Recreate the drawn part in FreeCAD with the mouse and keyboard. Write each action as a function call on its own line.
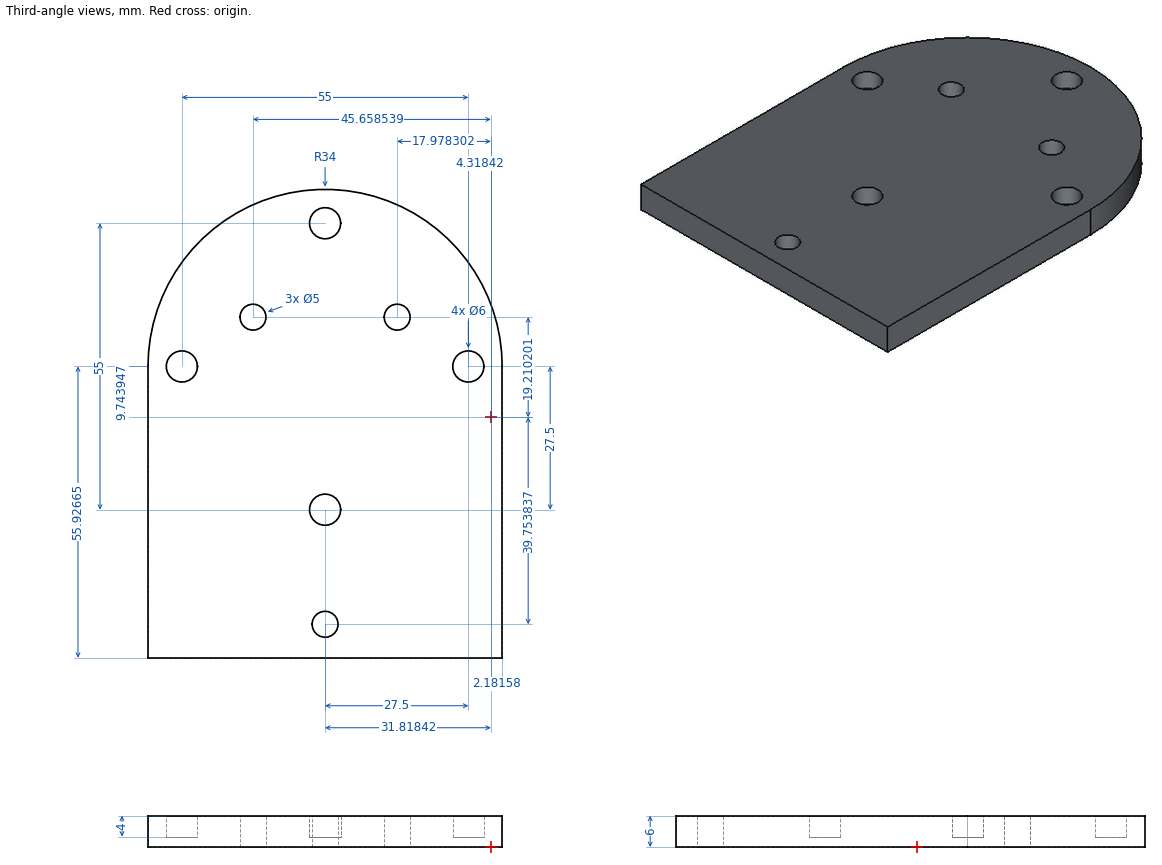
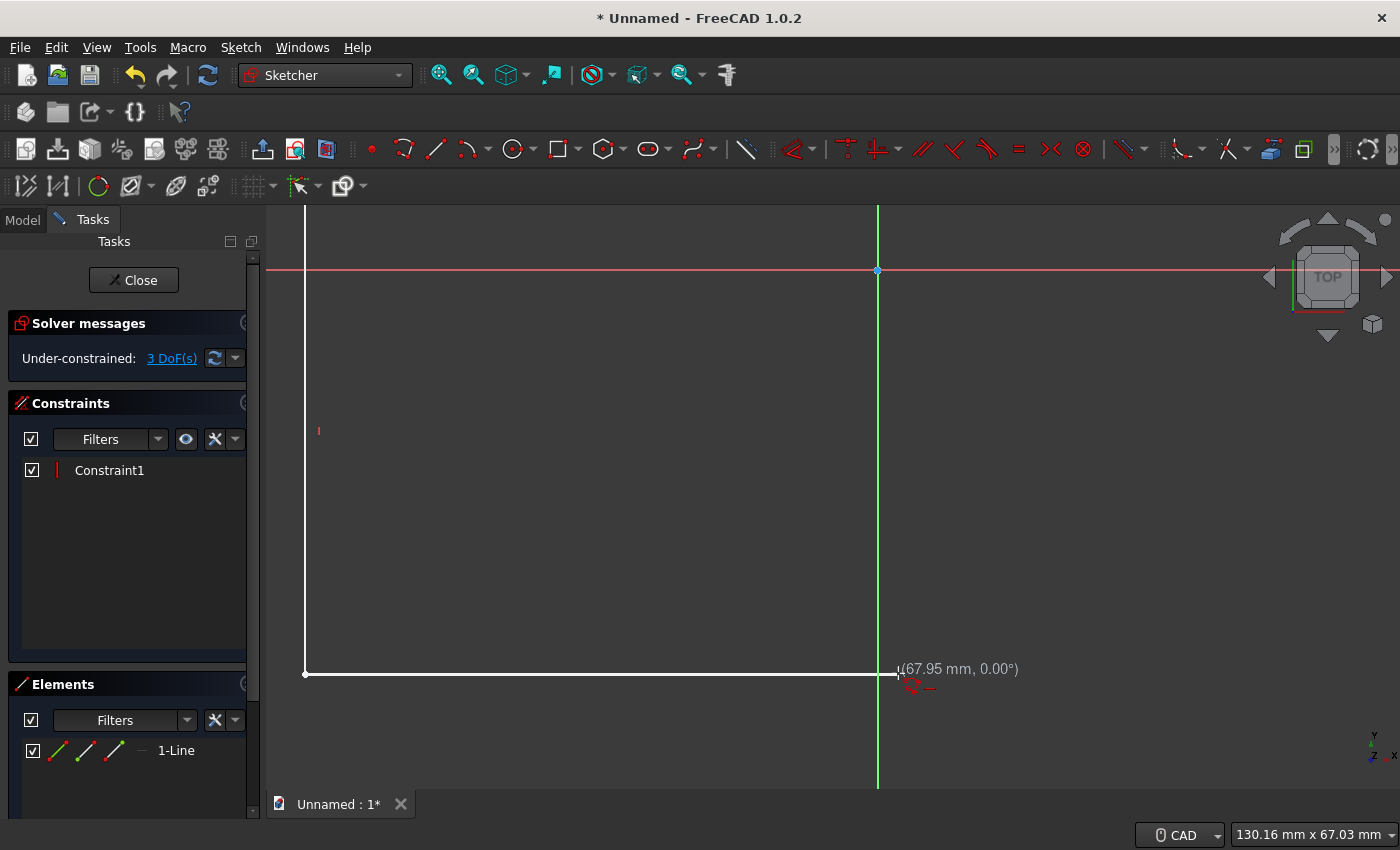
click(897, 672)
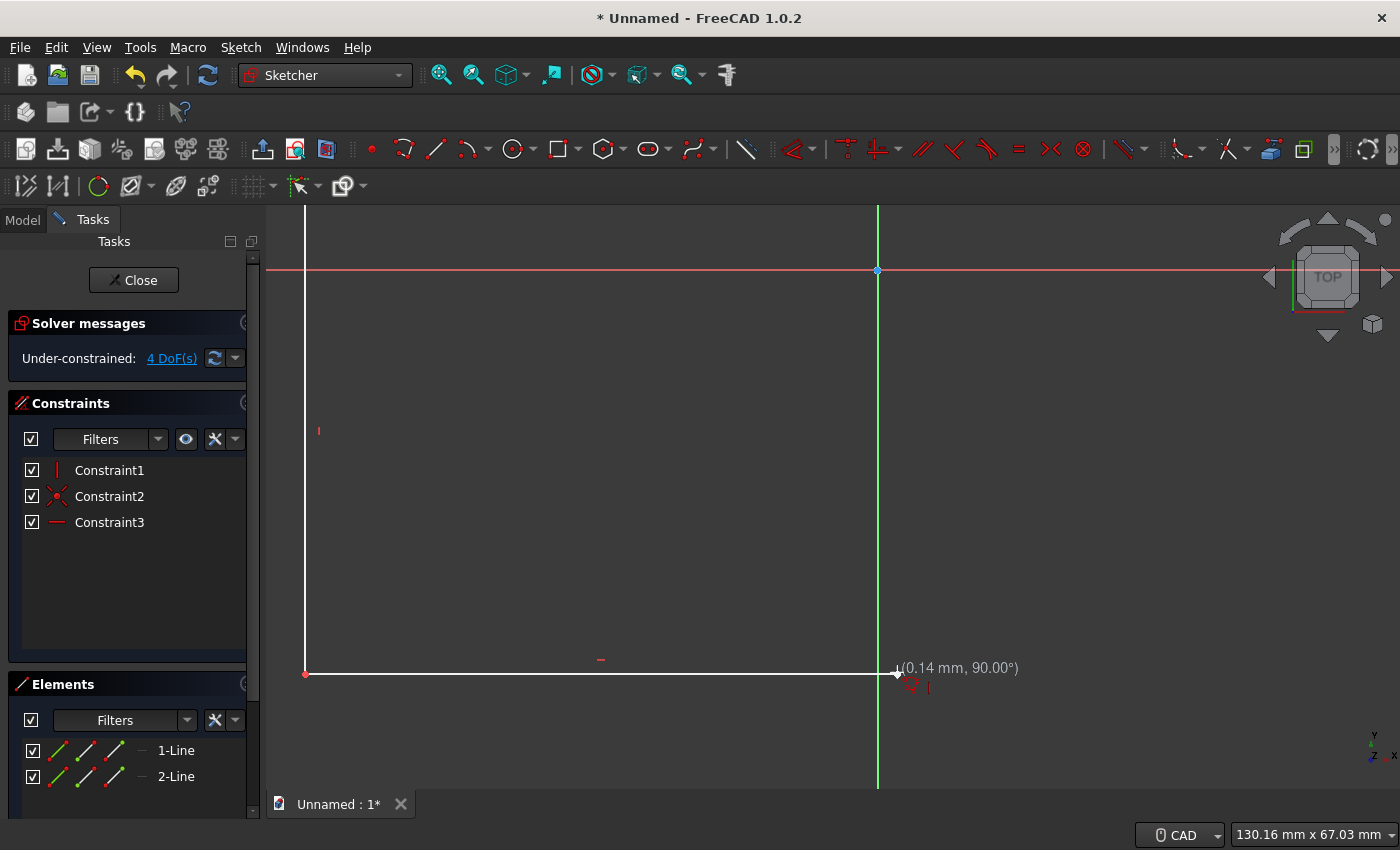
scroll(898, 673, down, 4)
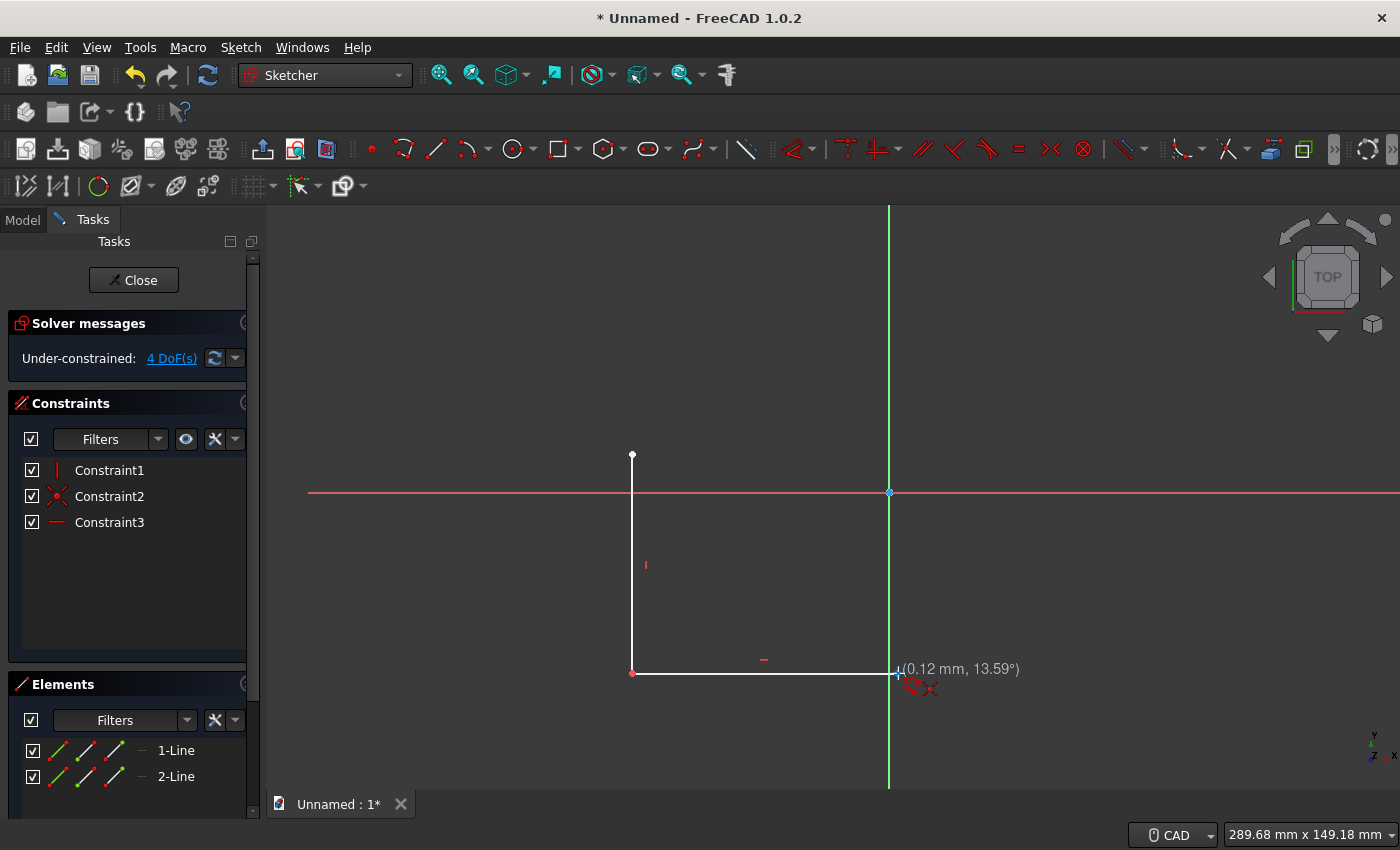
scroll(898, 454, up, 4)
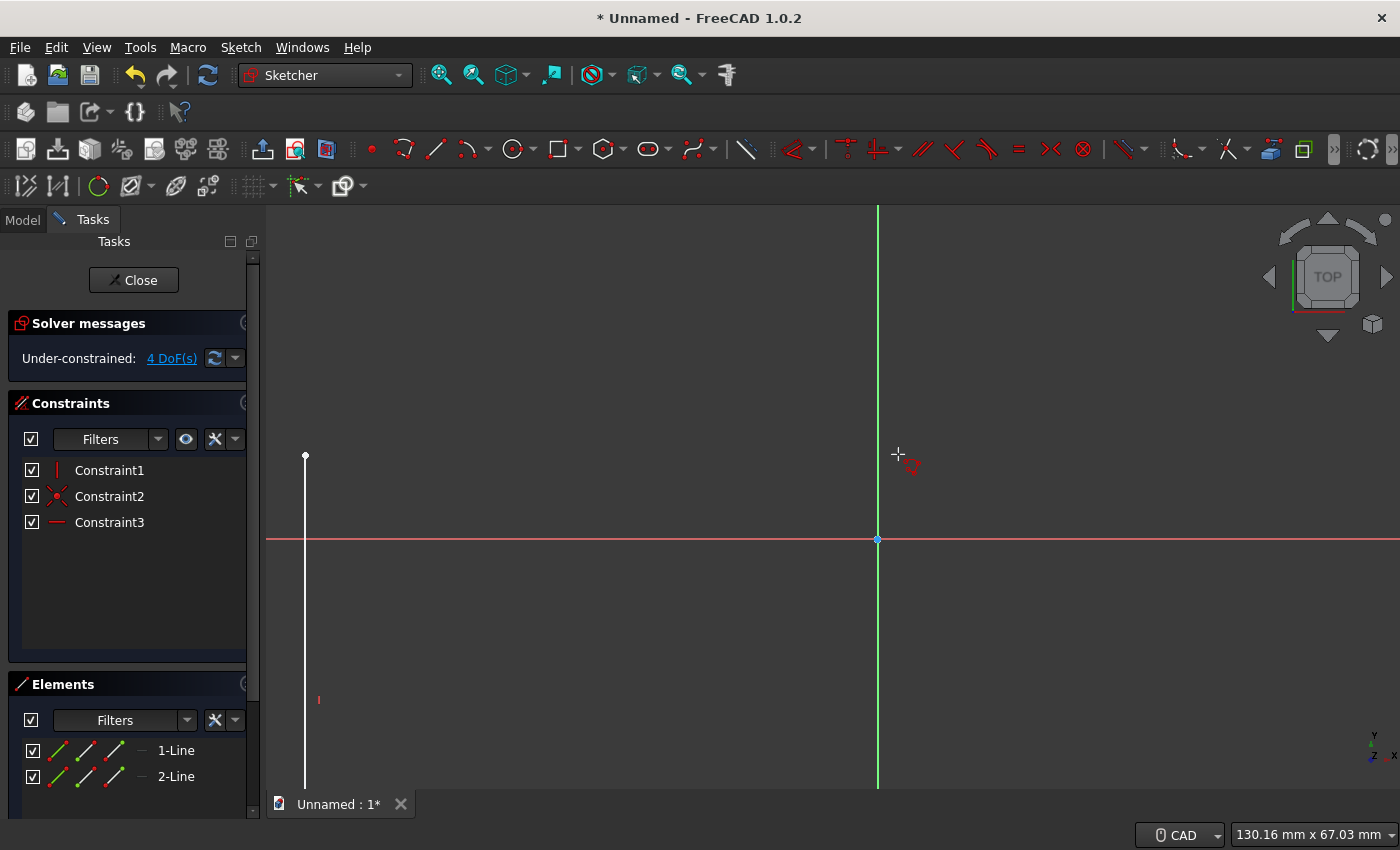
click(897, 454)
right_click(897, 454)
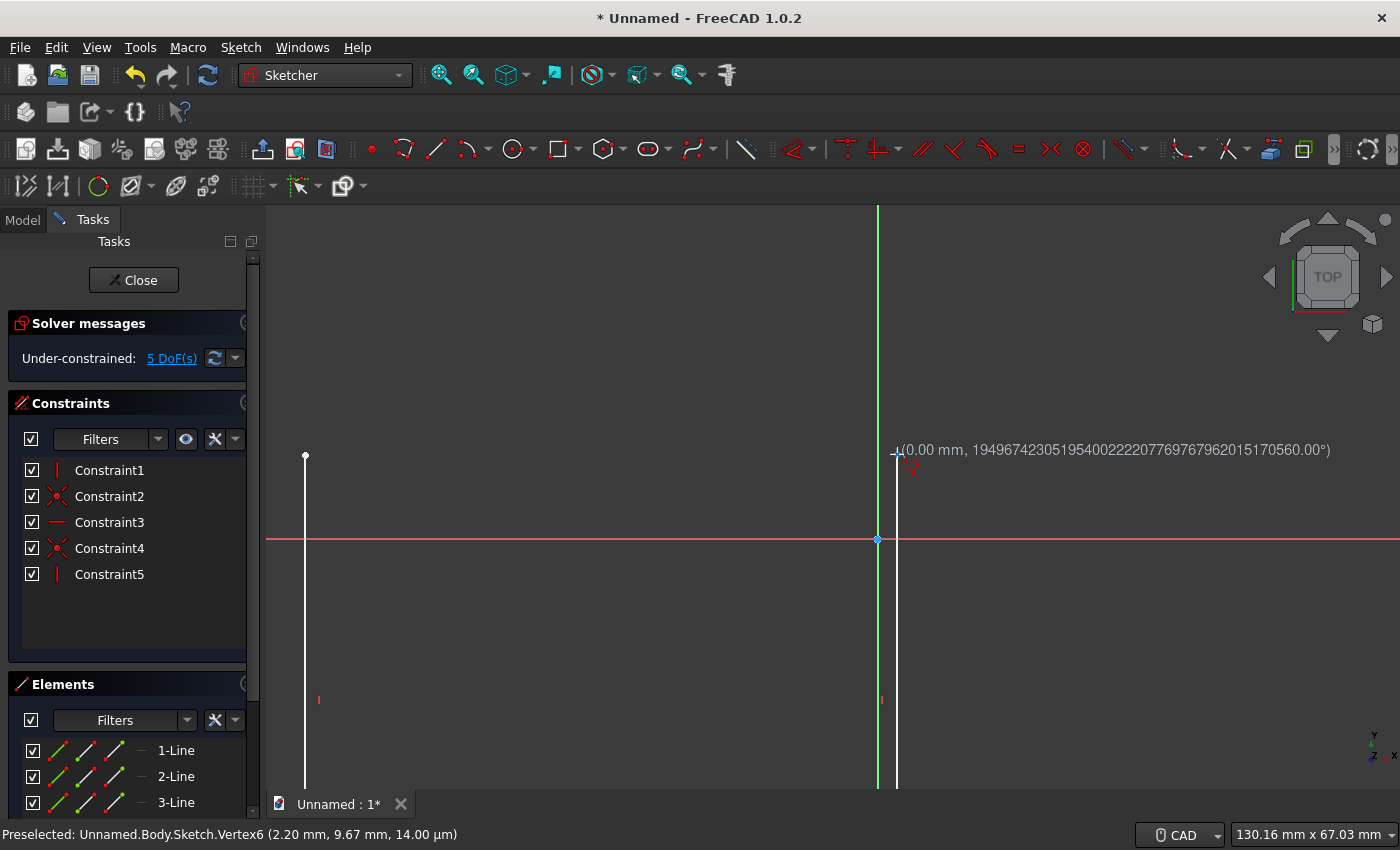
key(g)
key(3)
key(a)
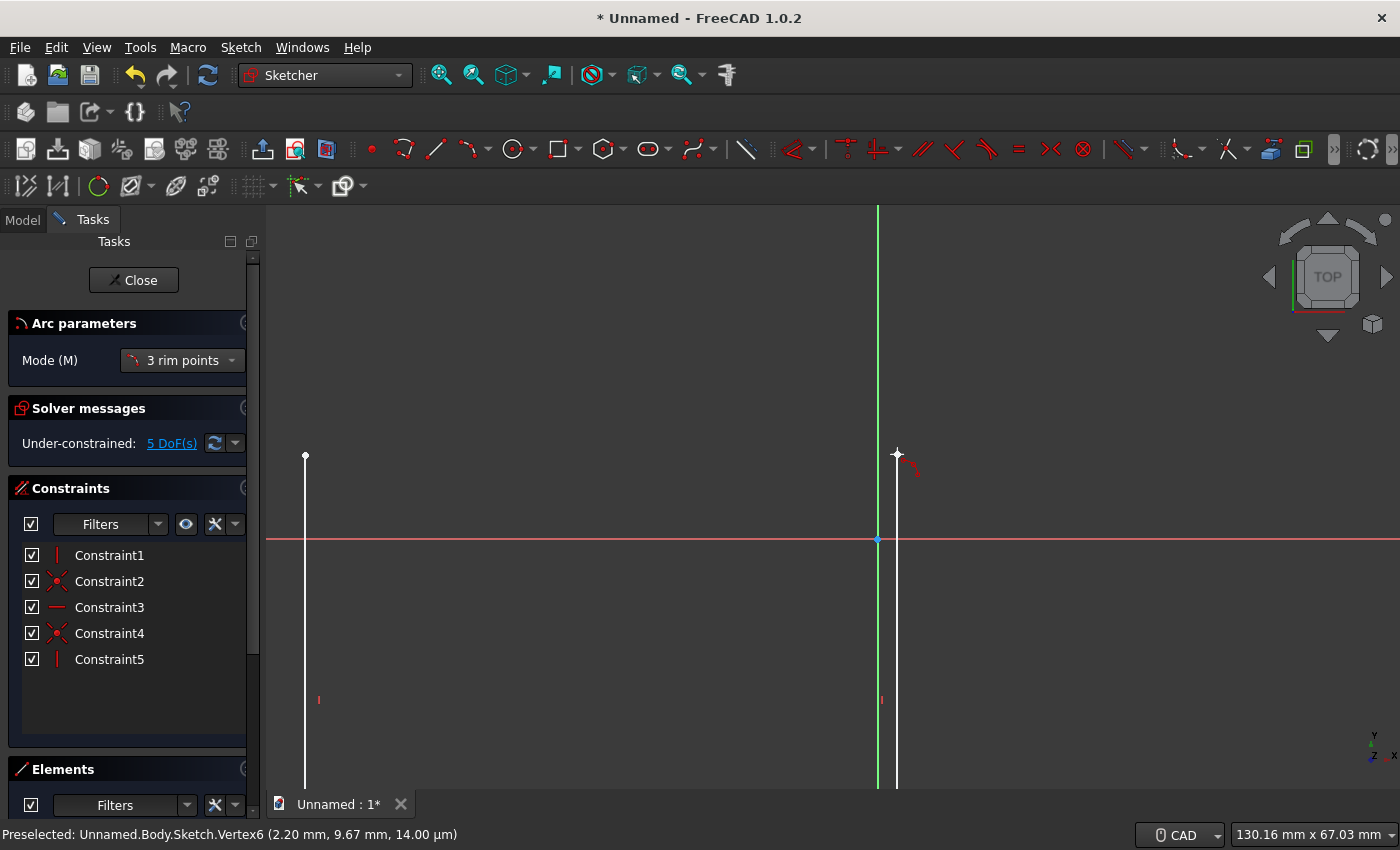
click(897, 455)
click(305, 456)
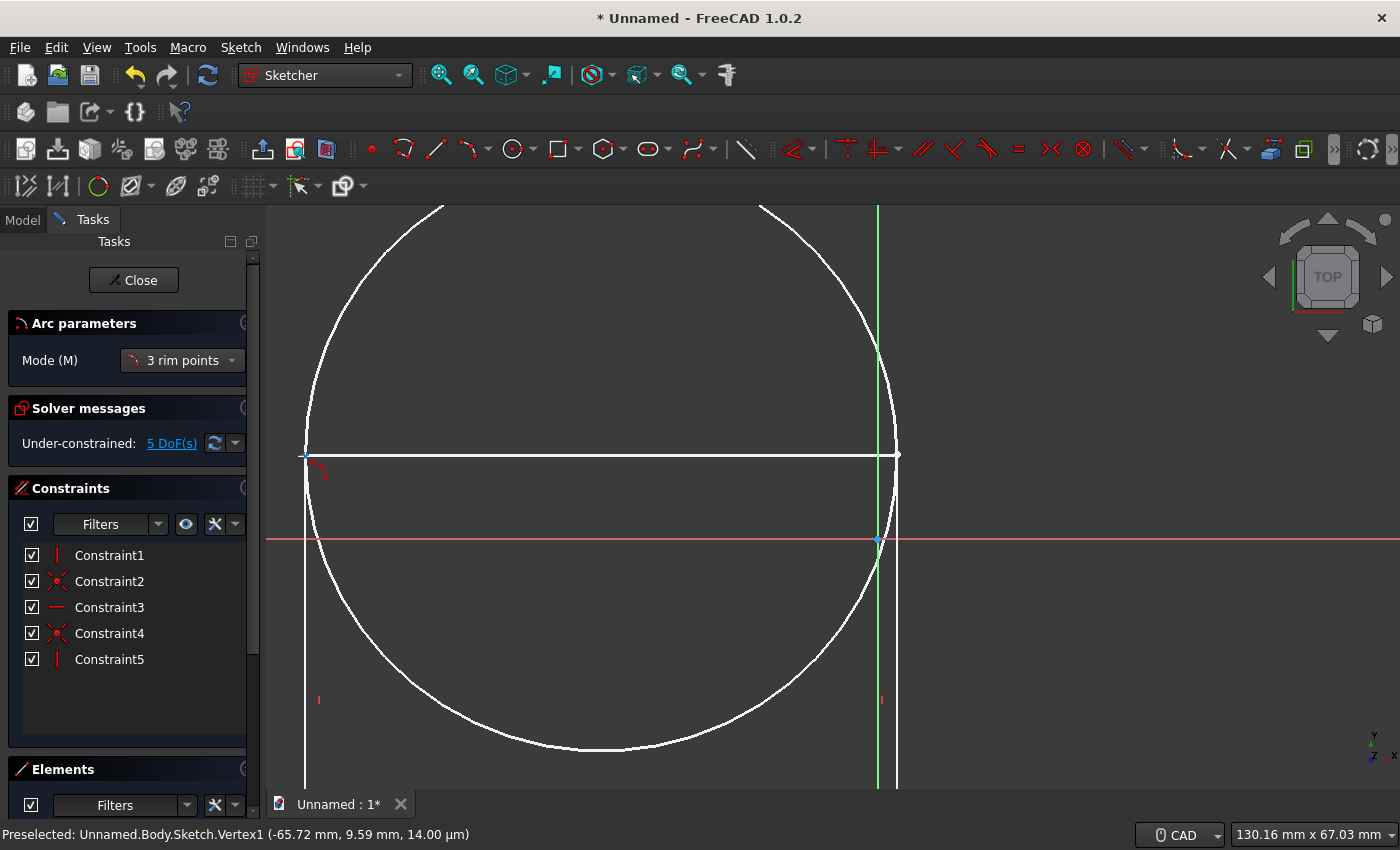
scroll(898, 454, down, 4)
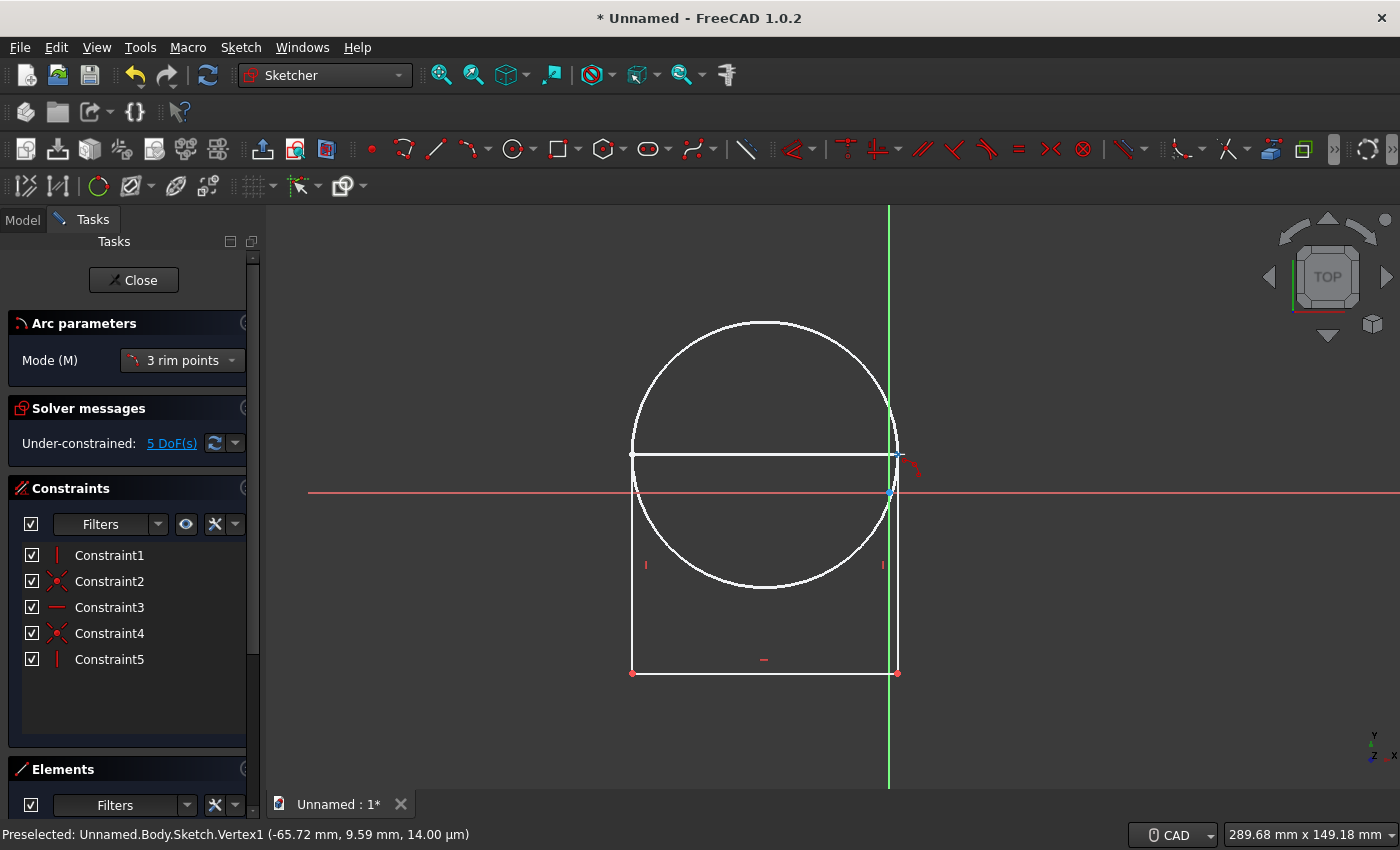
click(765, 321)
key(Escape)